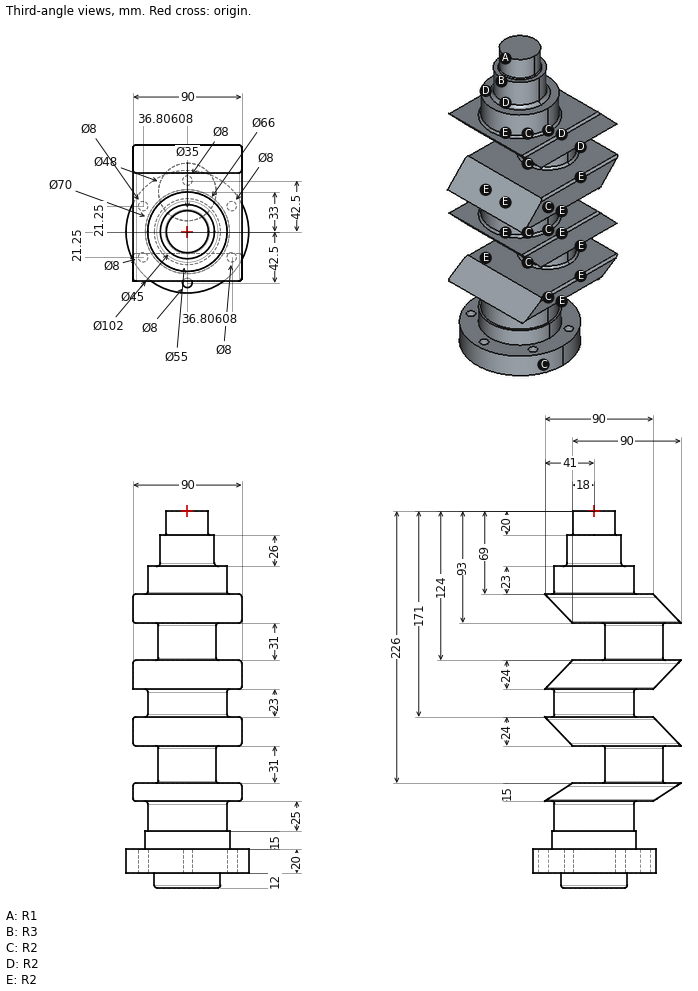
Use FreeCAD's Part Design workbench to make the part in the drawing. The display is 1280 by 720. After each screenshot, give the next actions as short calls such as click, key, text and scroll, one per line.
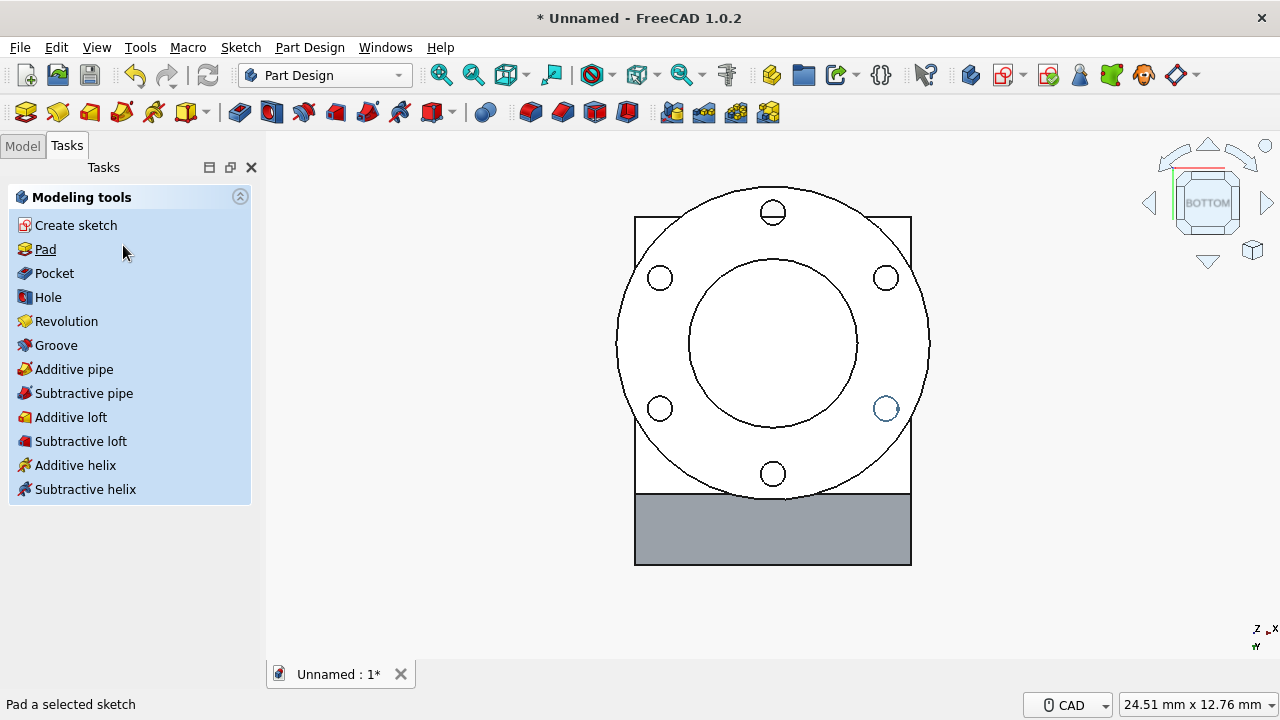
click(240, 112)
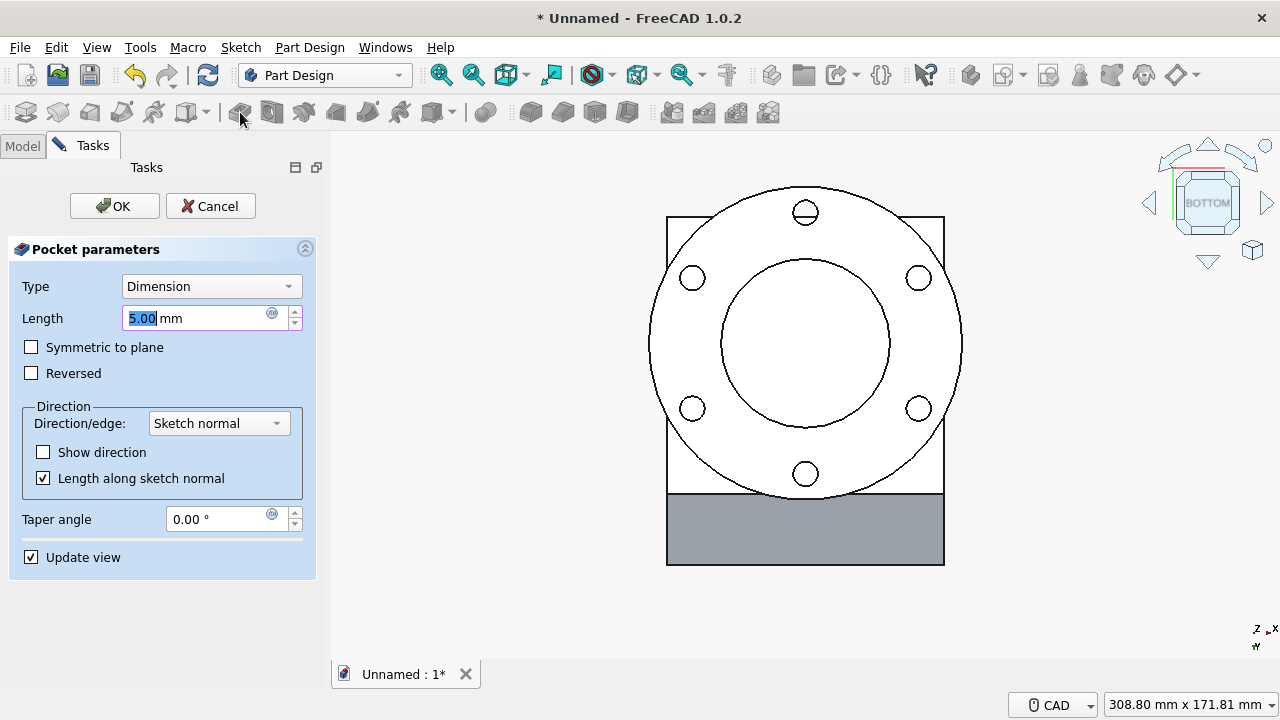
click(212, 286)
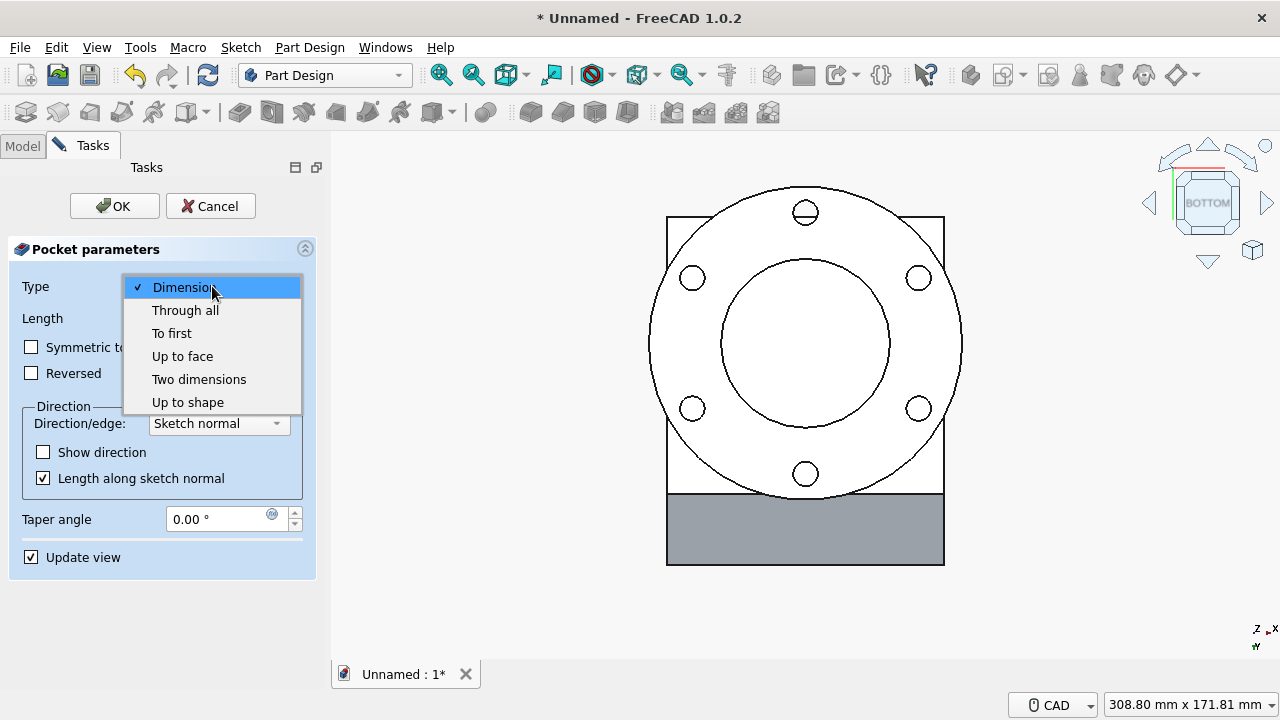
click(212, 334)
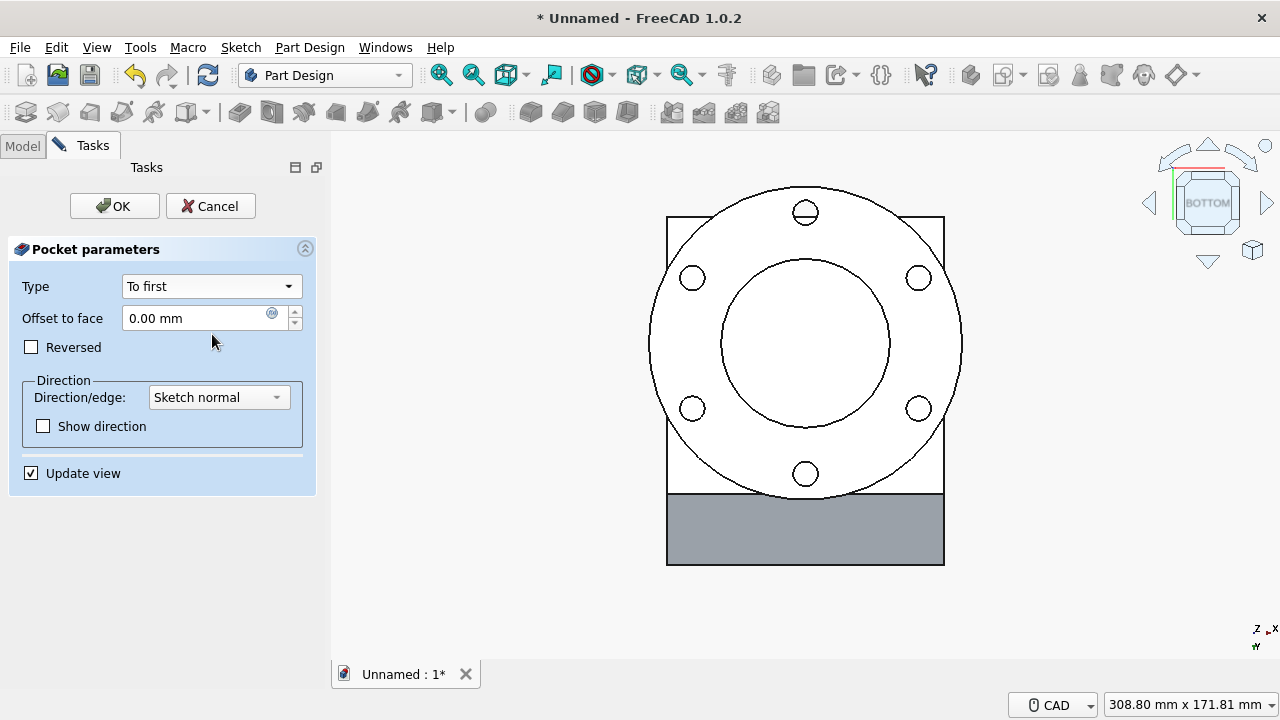
click(115, 206)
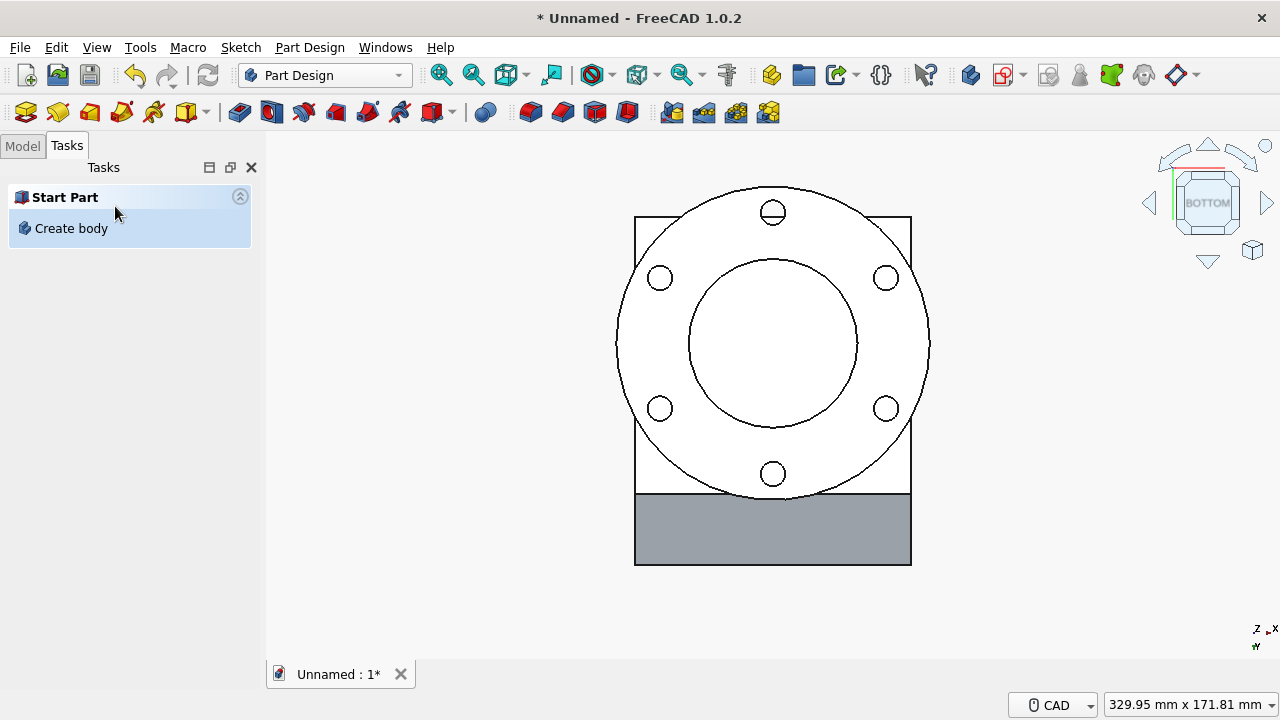
key(0)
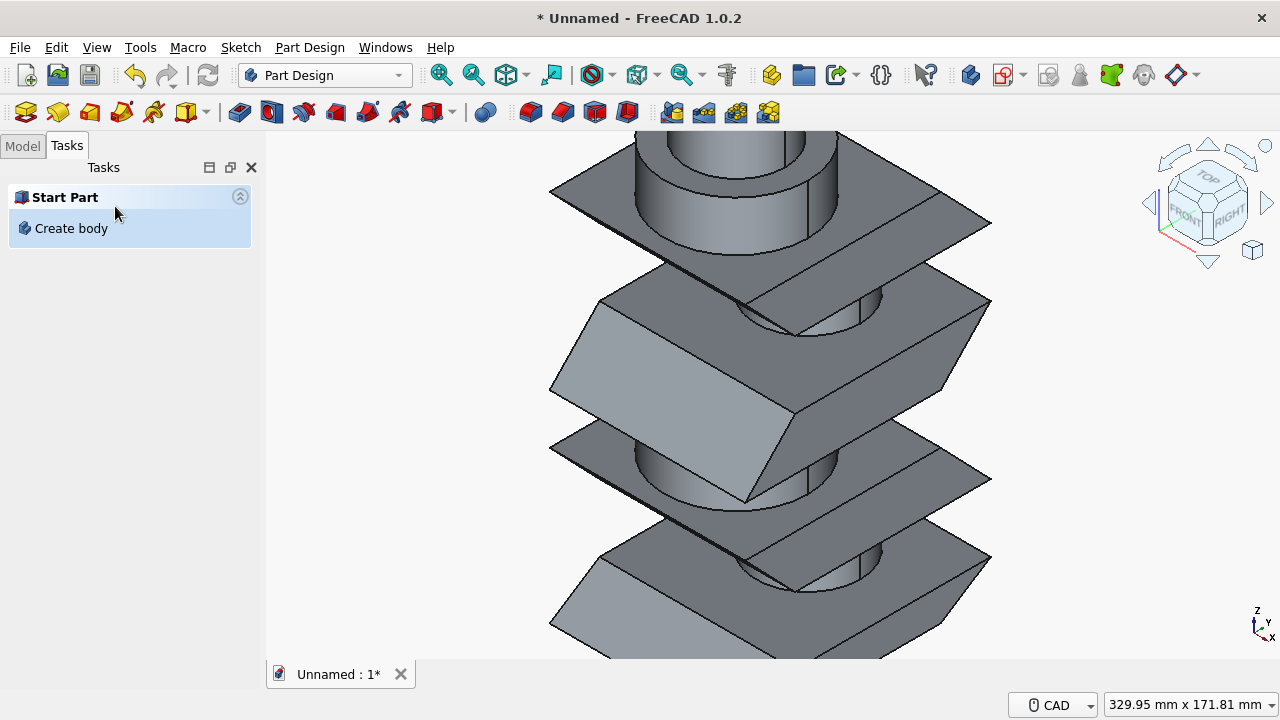
click(442, 76)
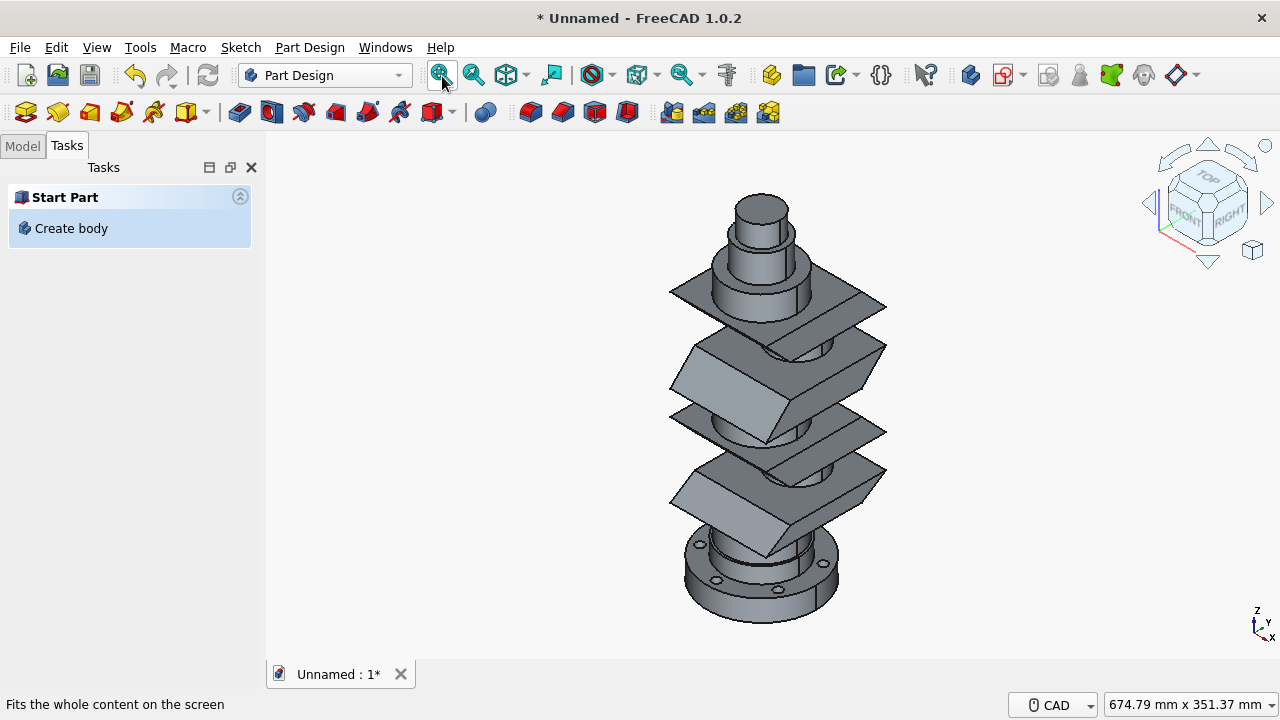
key(2)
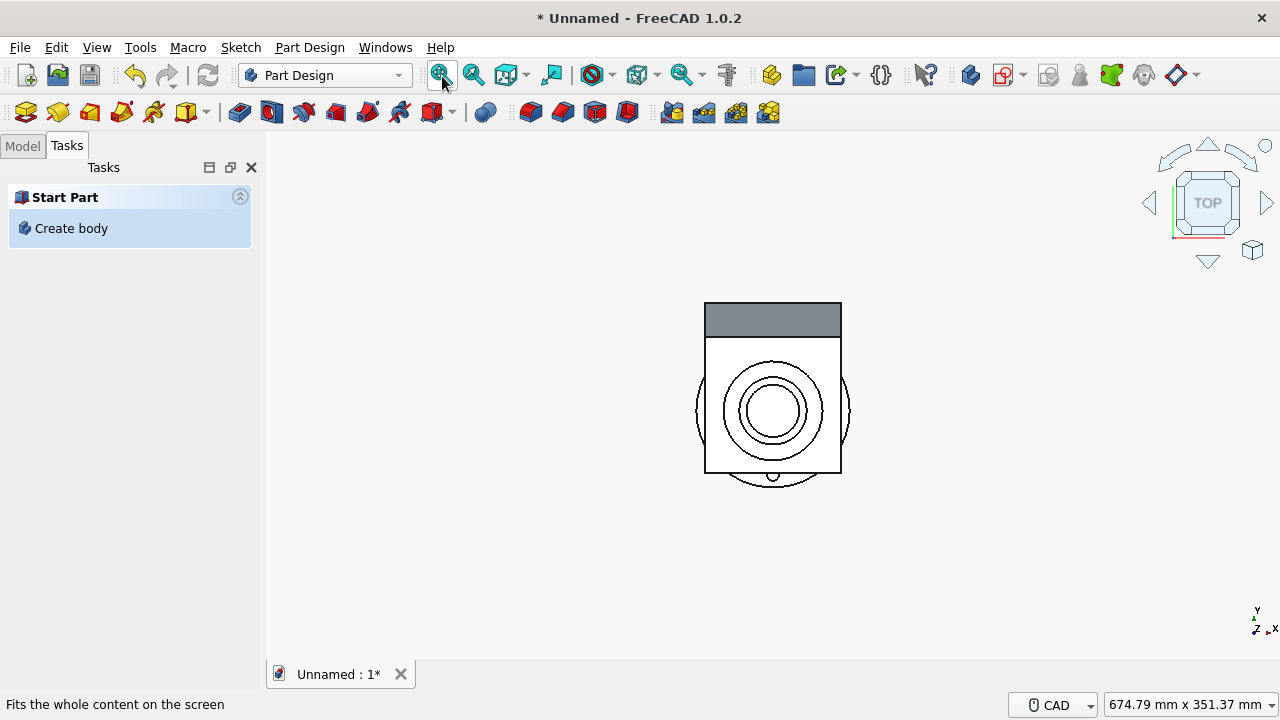
click(442, 76)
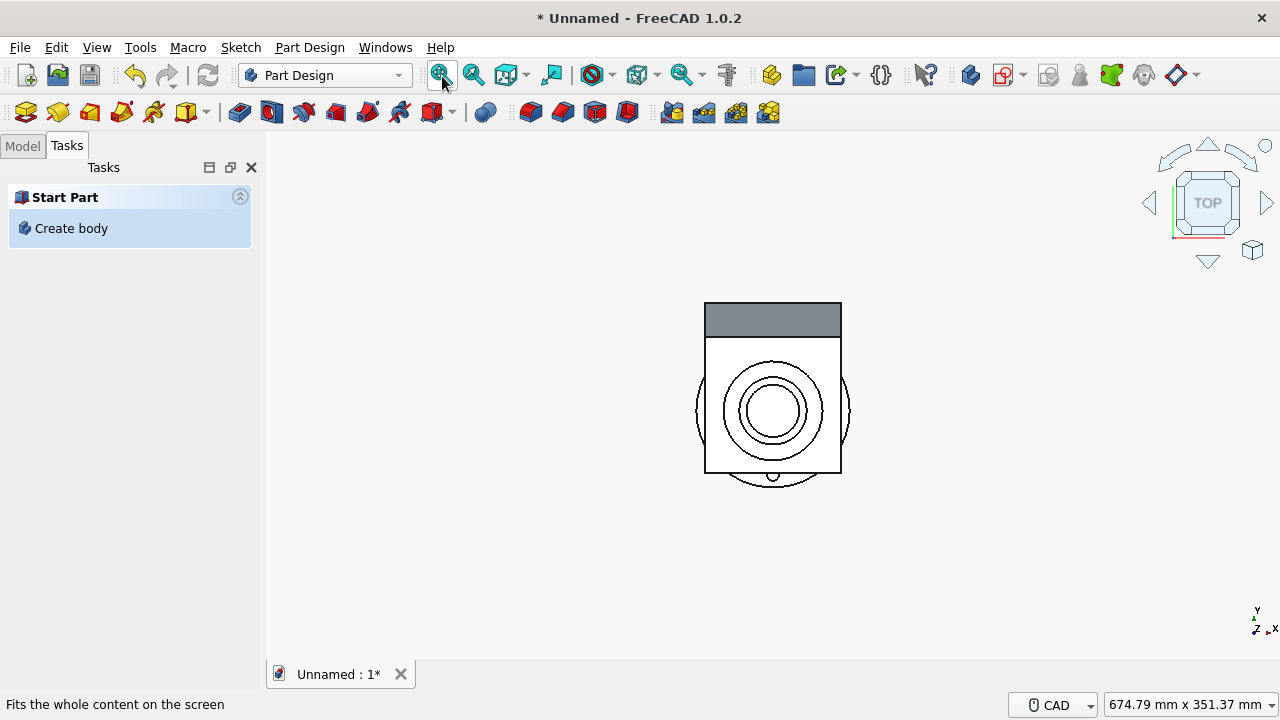
key(1)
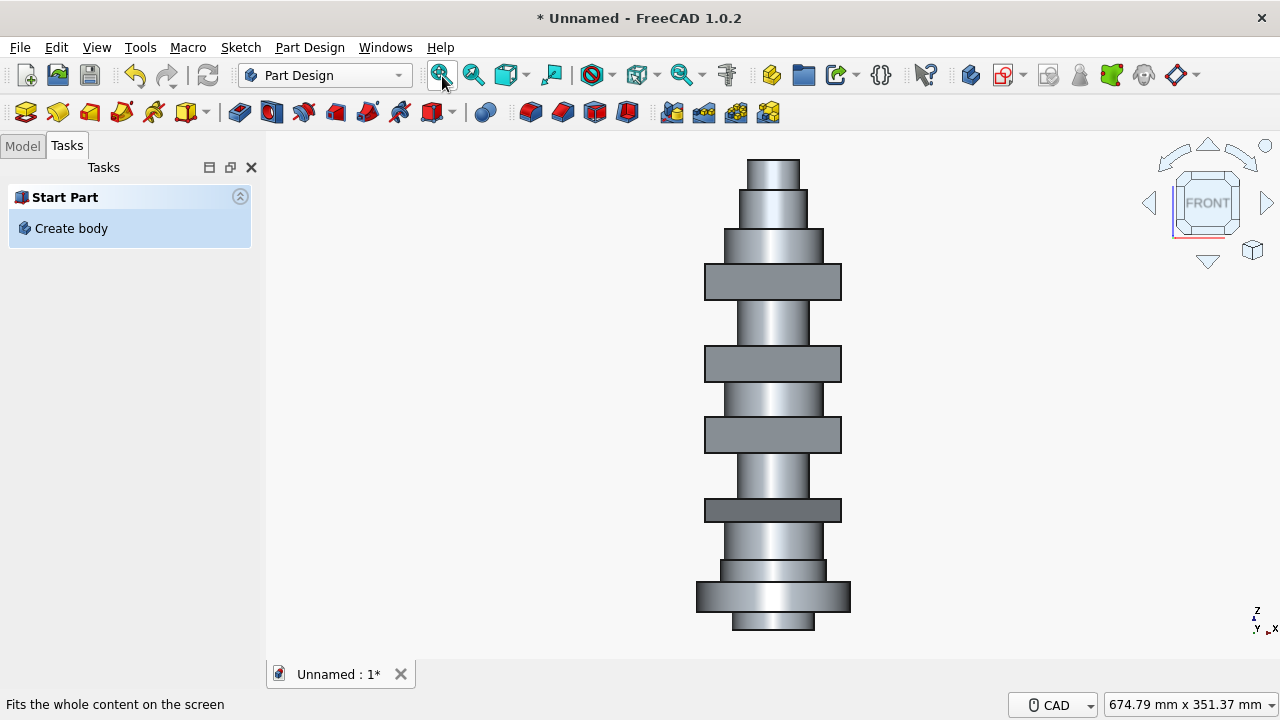
key(3)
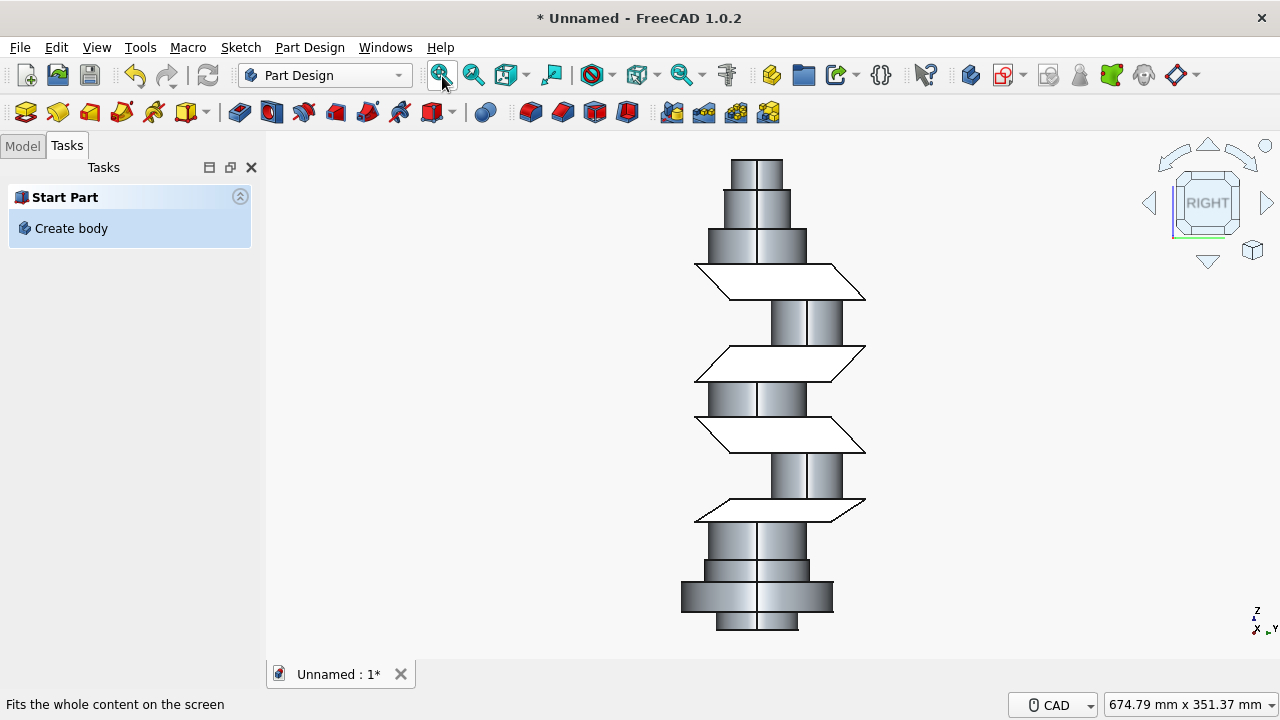
key(5)